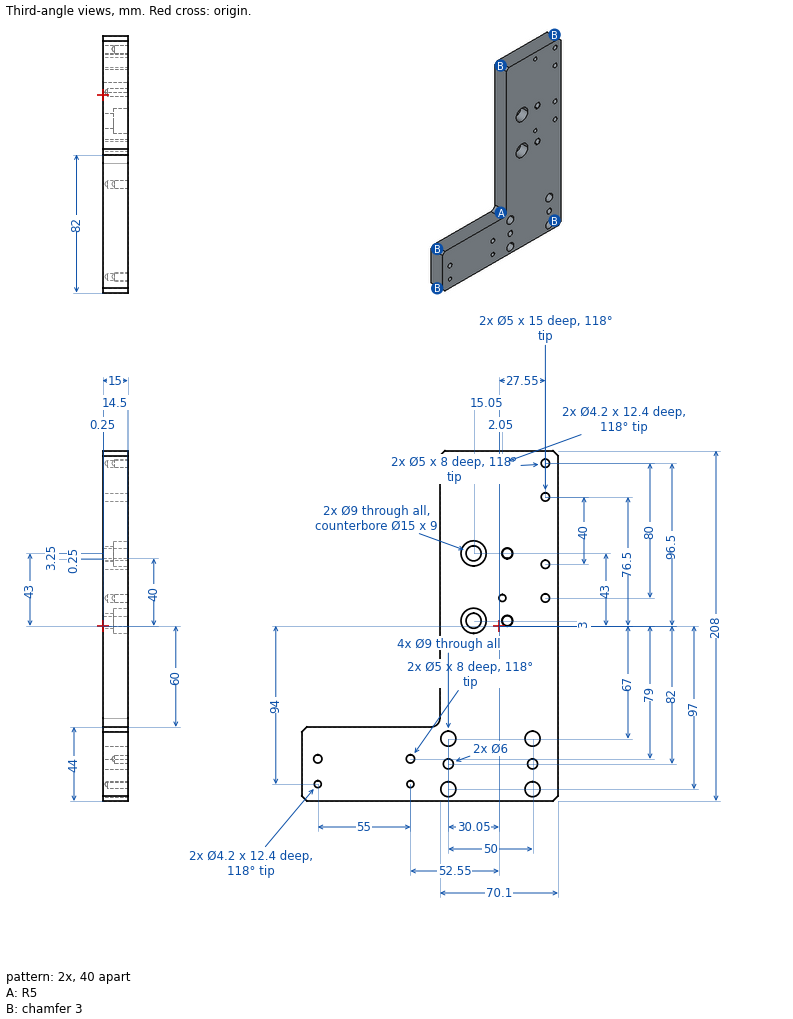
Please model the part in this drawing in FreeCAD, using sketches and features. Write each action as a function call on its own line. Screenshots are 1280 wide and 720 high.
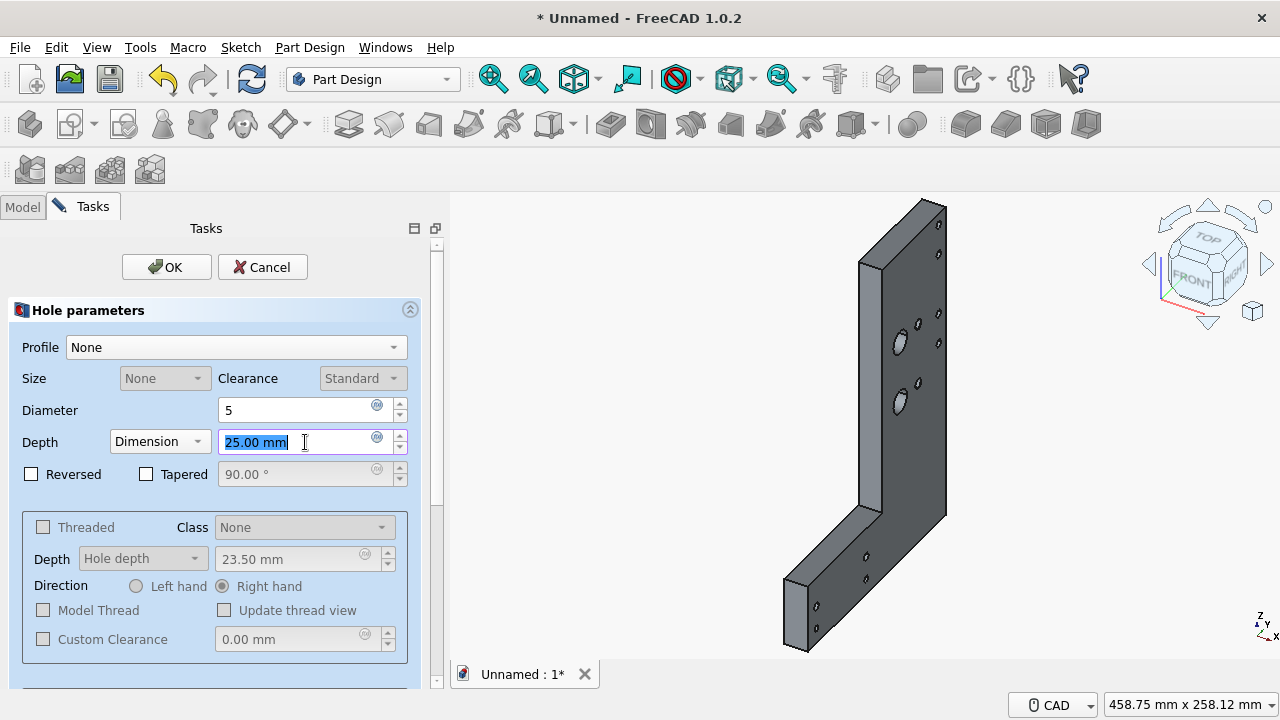
text(8)
key(Tab)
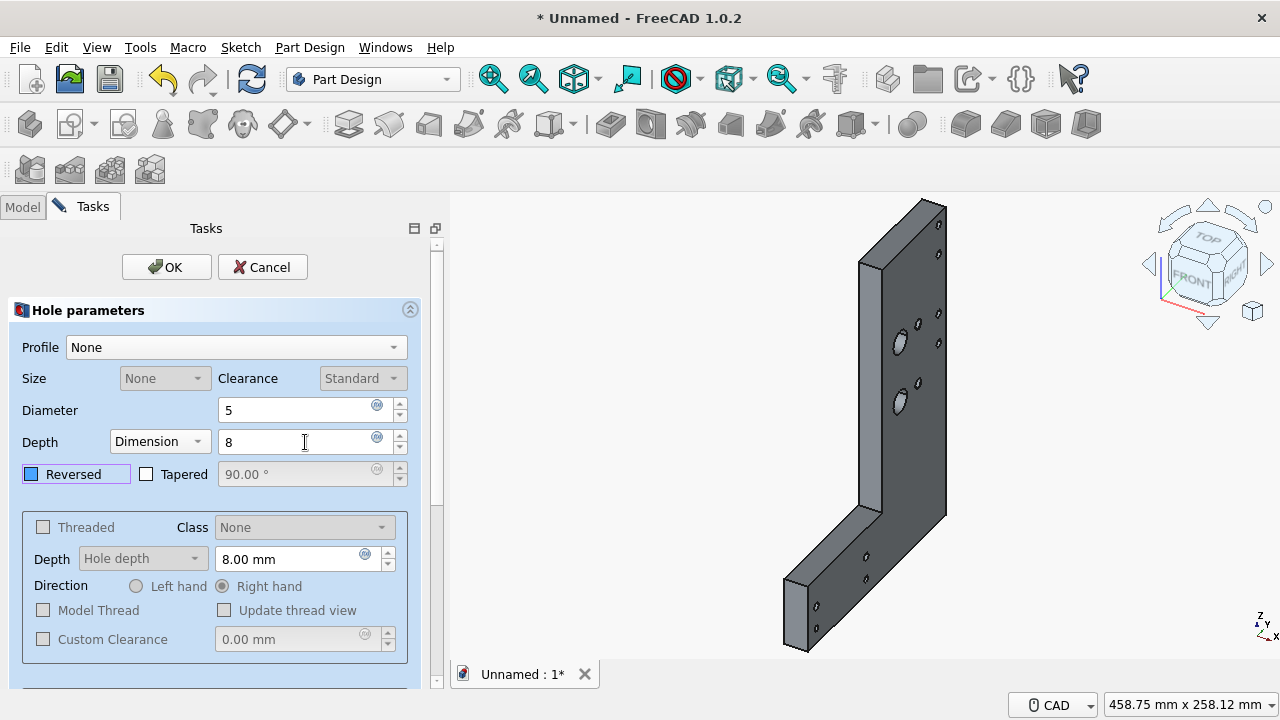
click(167, 267)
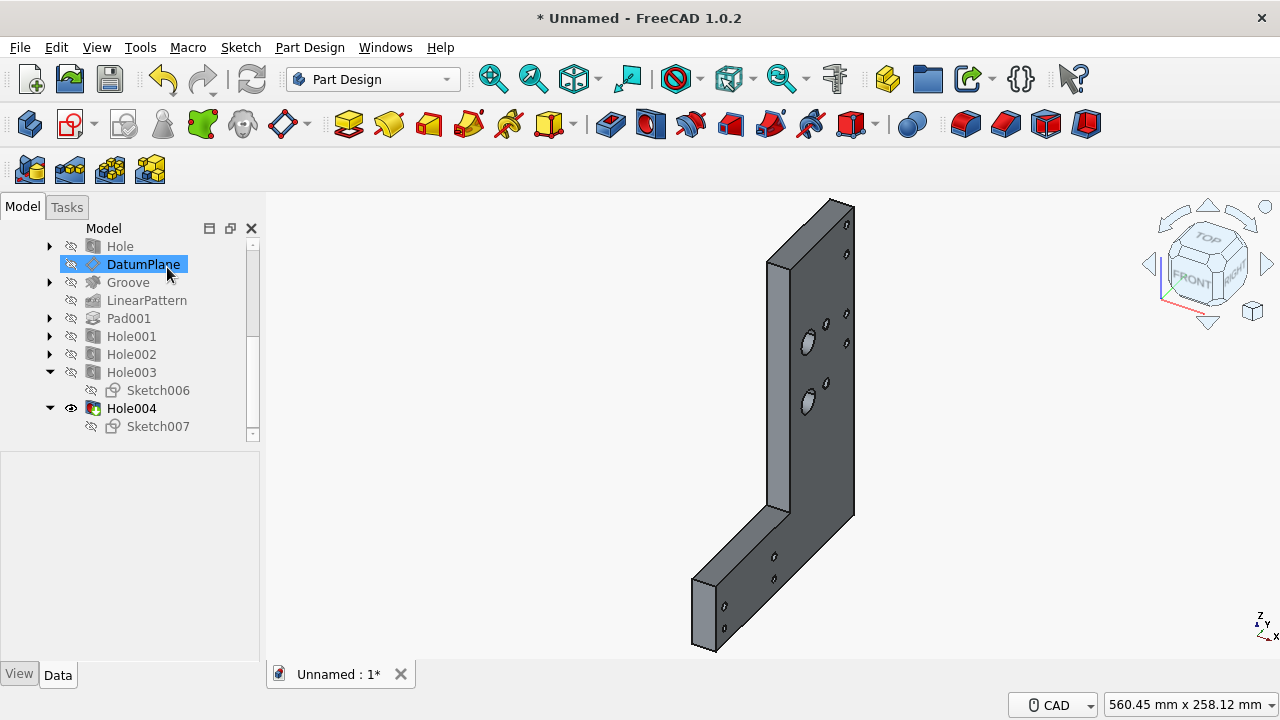
click(824, 477)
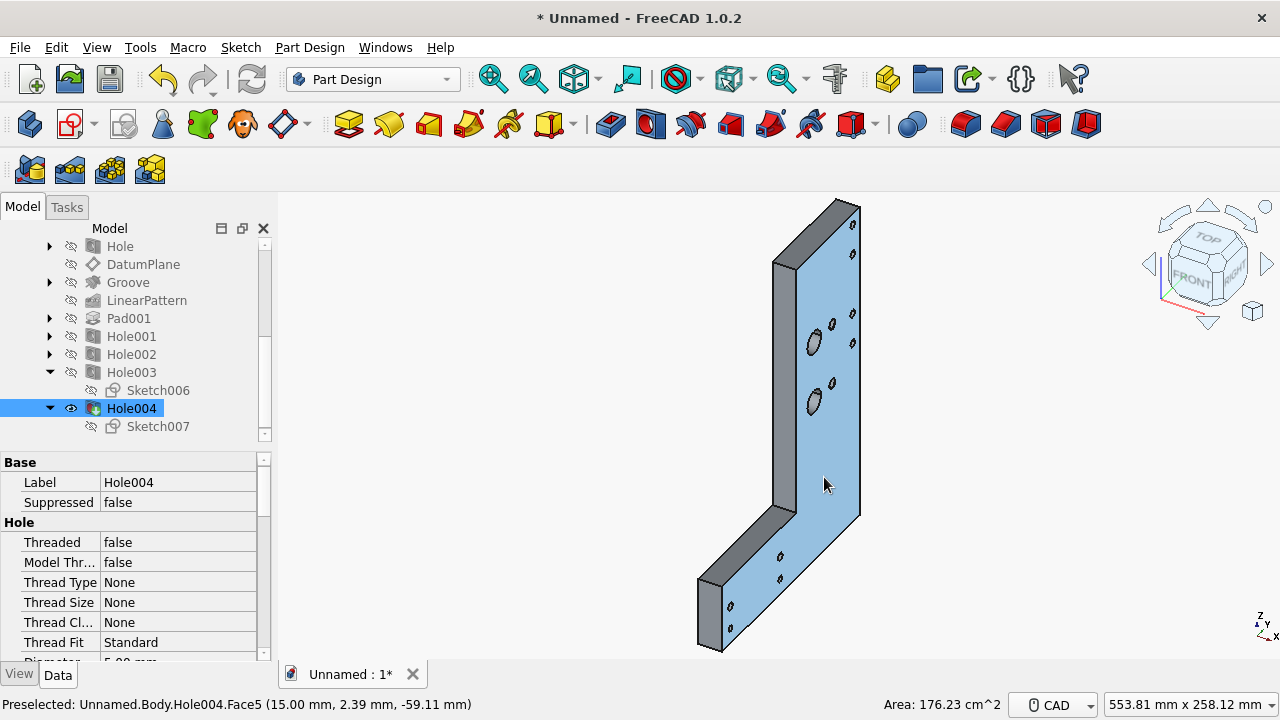
click(70, 124)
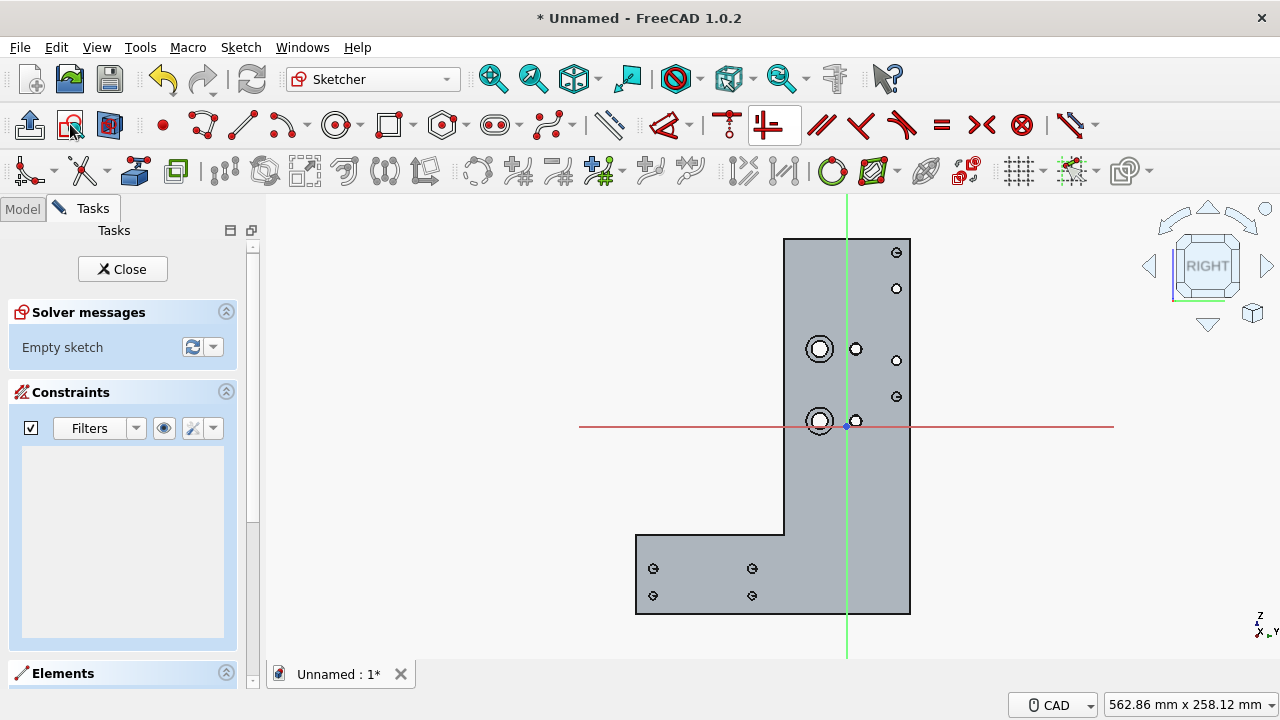
scroll(1115, 222, up, 2)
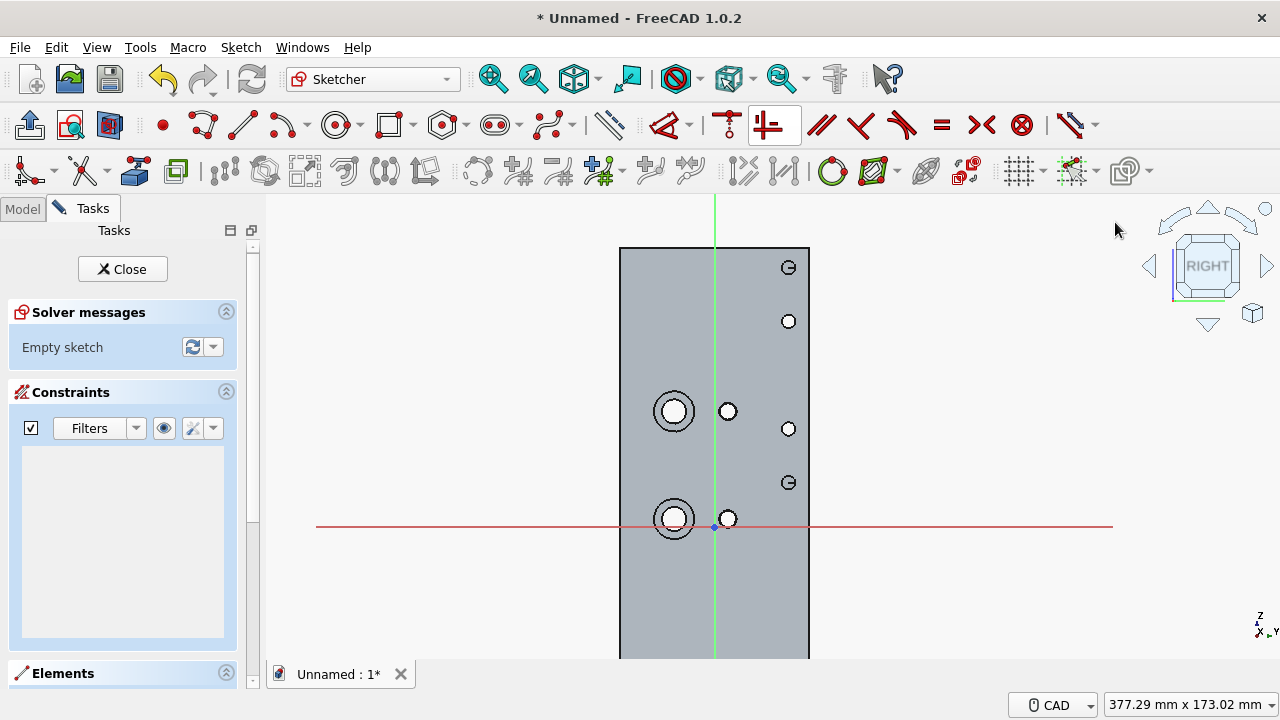
key(g)
key(c)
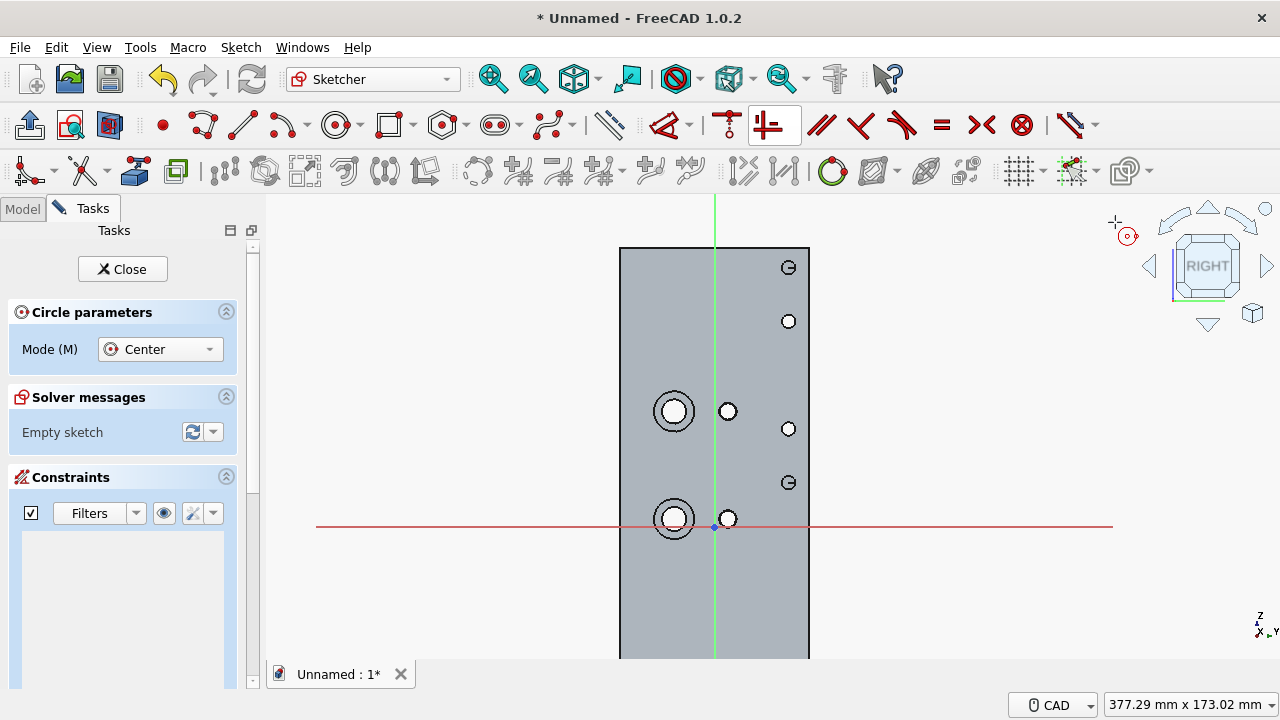
scroll(720, 268, up, 7)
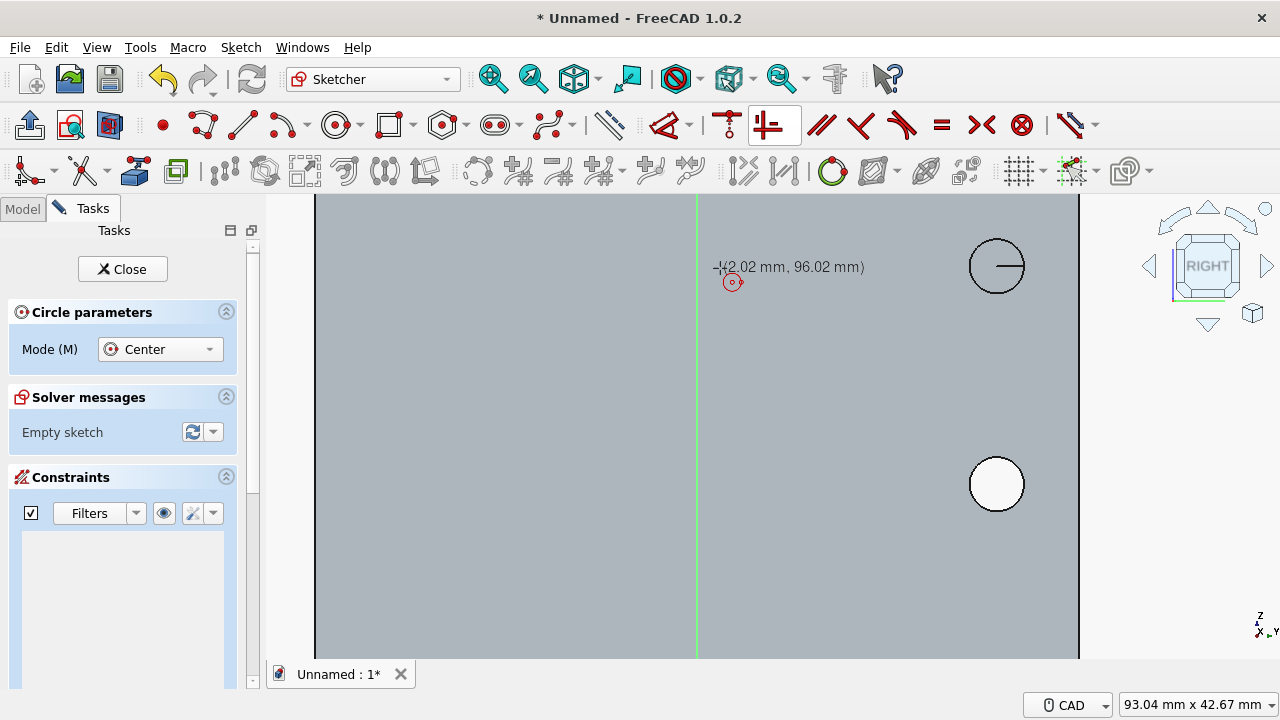
click(719, 266)
click(735, 250)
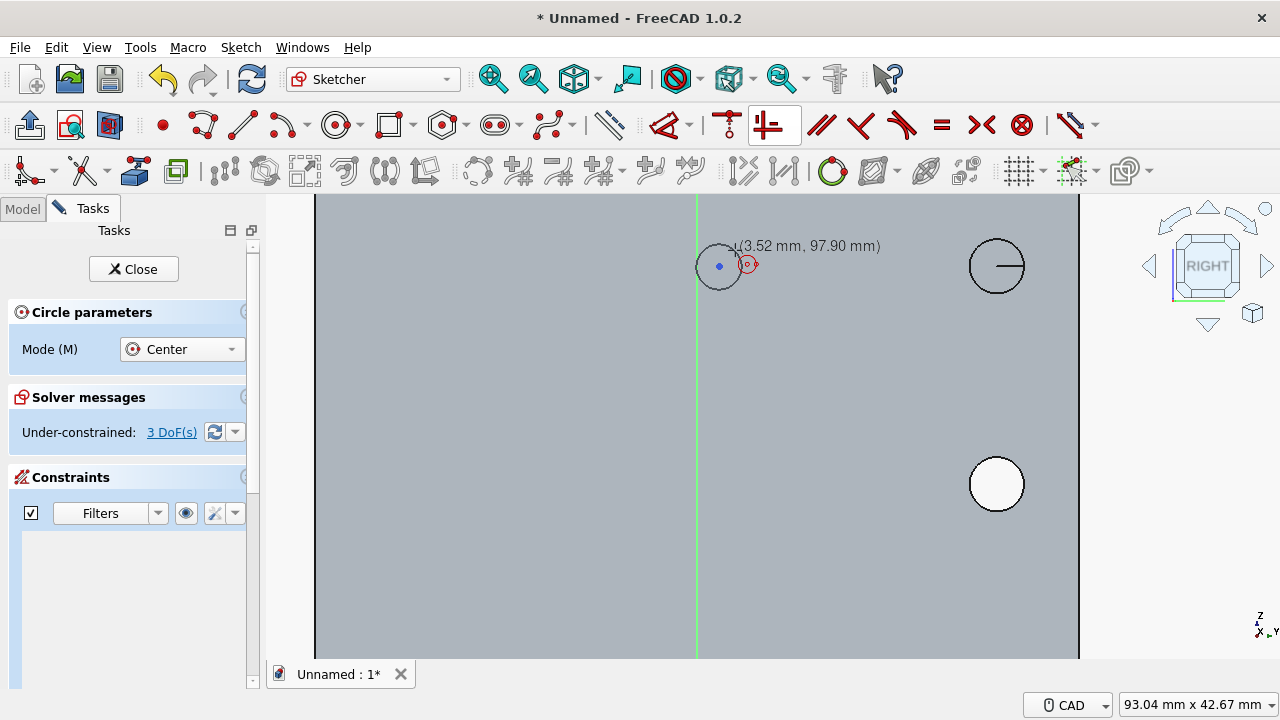
scroll(700, 311, down, 7)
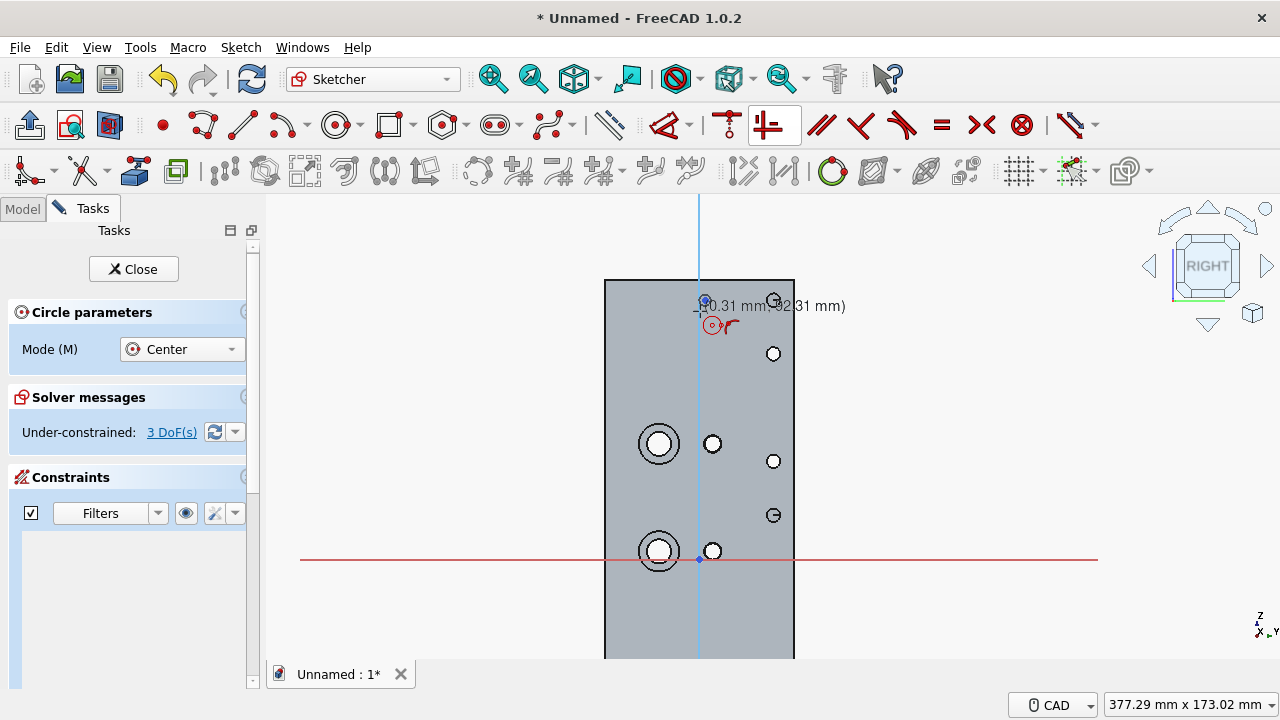
scroll(705, 515, up, 7)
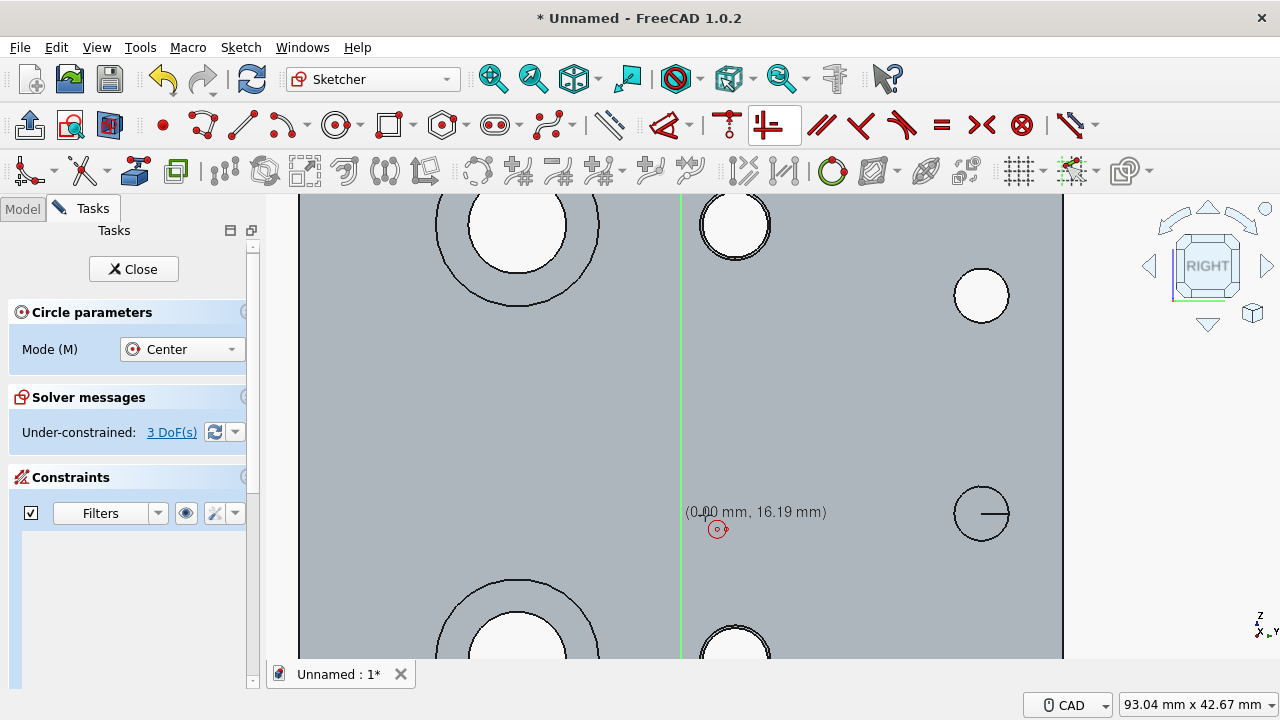
click(704, 514)
click(720, 497)
key(Escape)